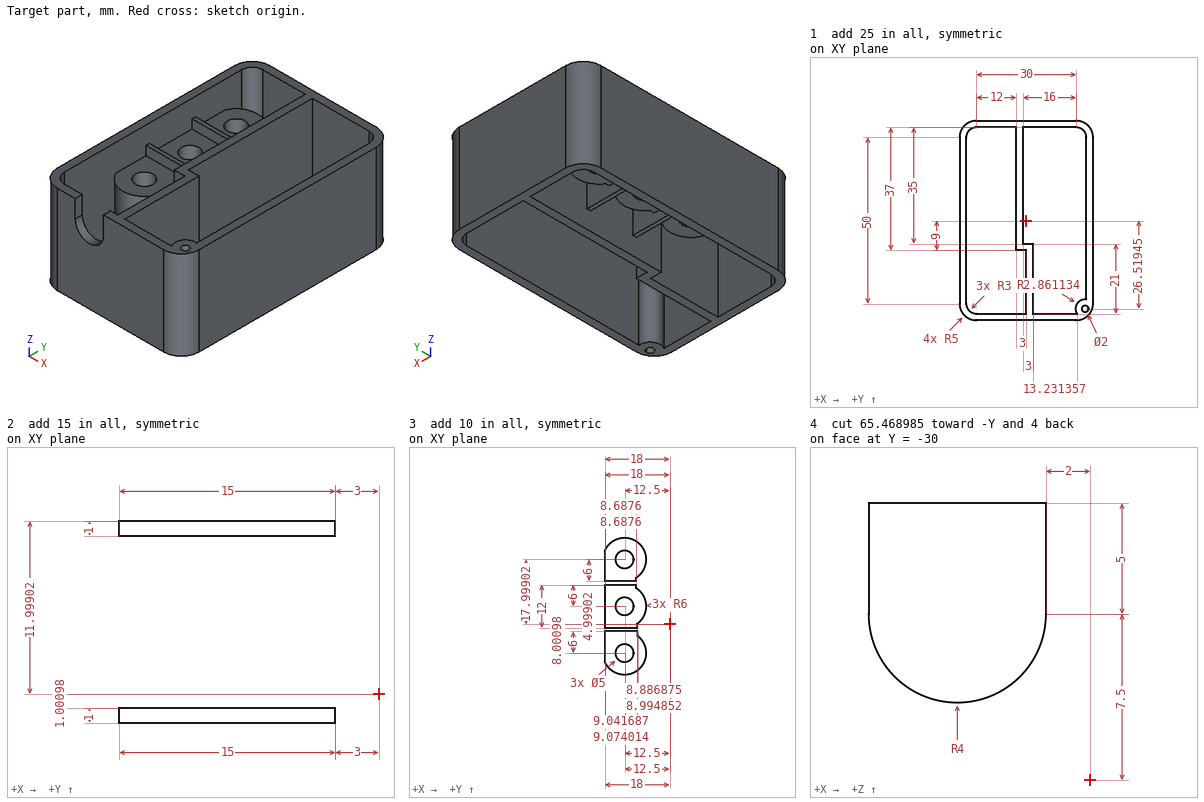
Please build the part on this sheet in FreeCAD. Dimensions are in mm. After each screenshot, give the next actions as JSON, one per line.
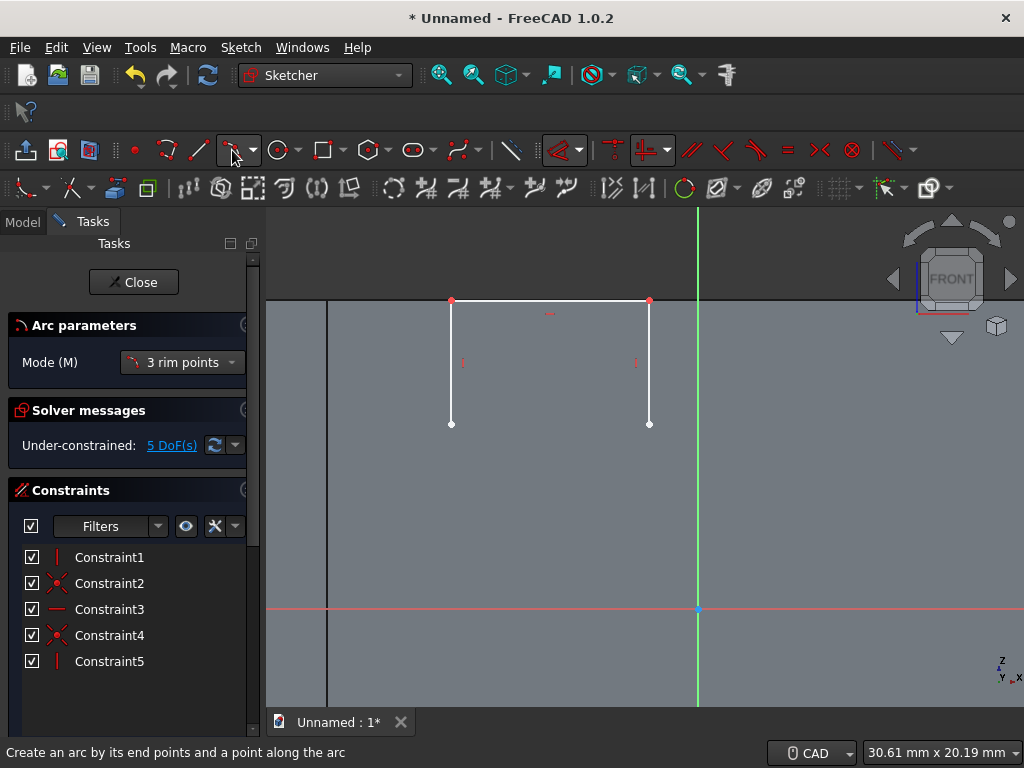
{"action": "left_click", "coordinate": [451, 425]}
{"action": "left_click", "coordinate": [649, 425]}
{"action": "left_click", "coordinate": [550, 523]}
{"action": "key", "text": "Escape"}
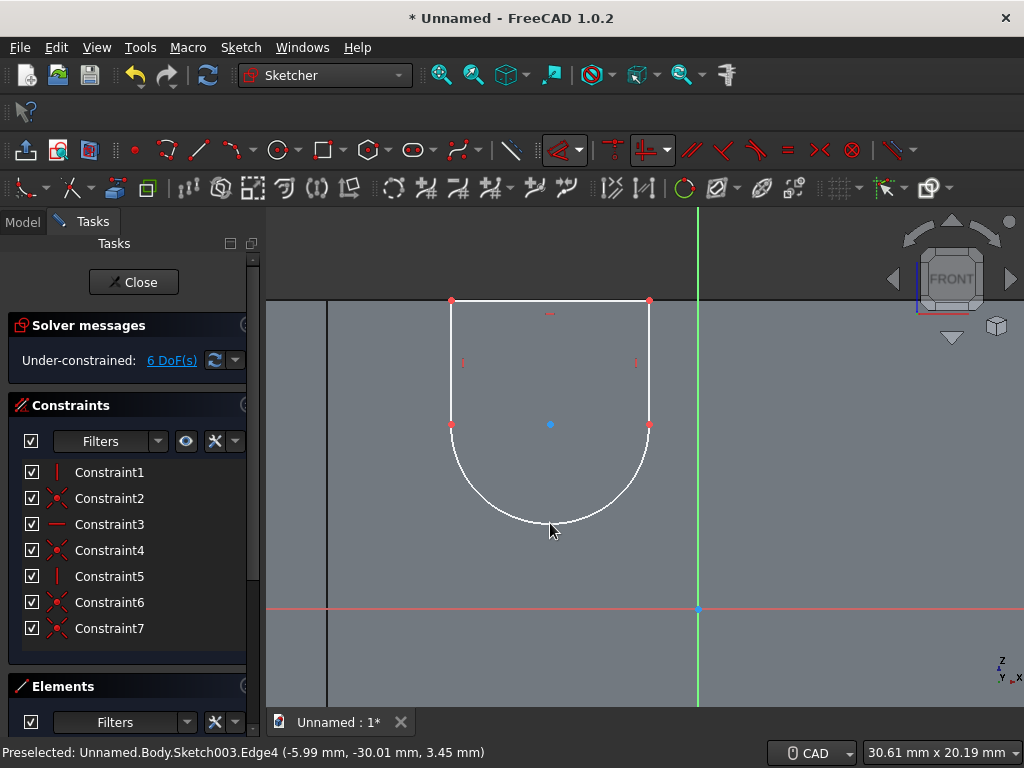
{"action": "left_click", "coordinate": [649, 388]}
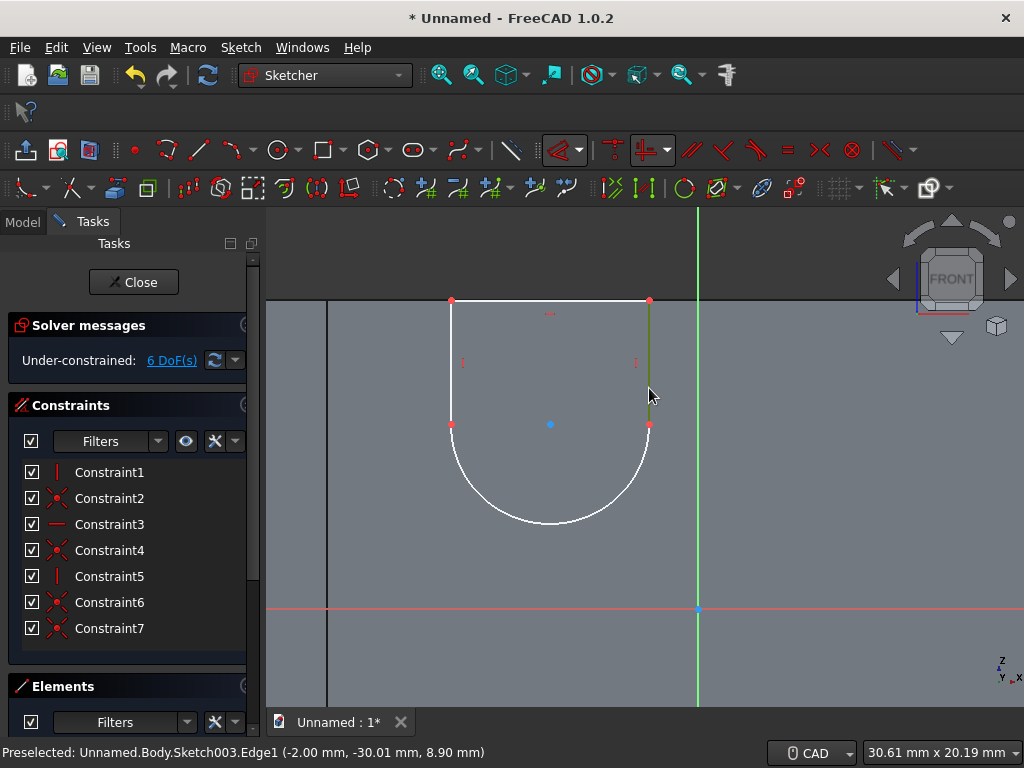
{"action": "left_click", "coordinate": [492, 505]}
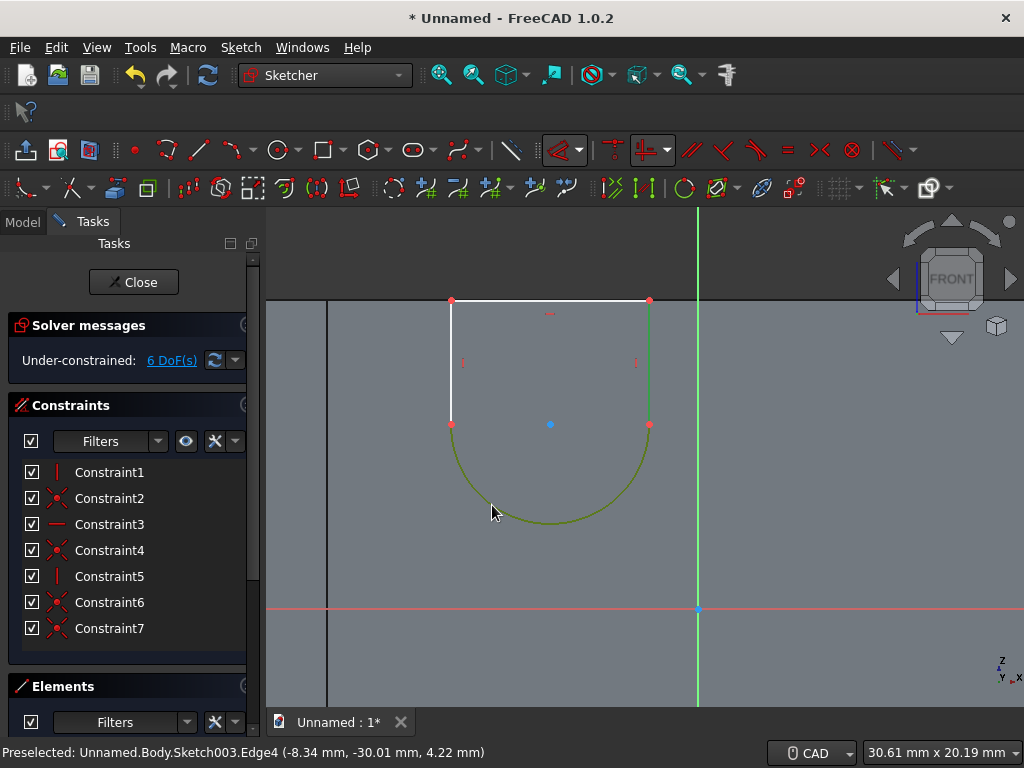
{"action": "left_click", "coordinate": [756, 150]}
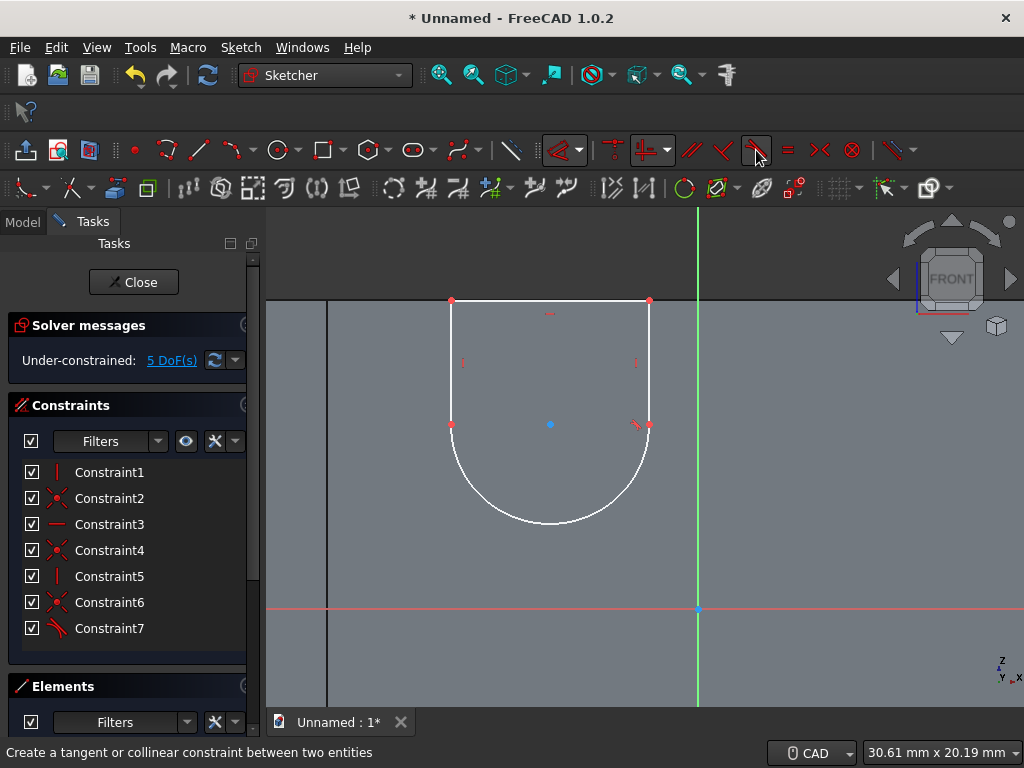
{"action": "left_click", "coordinate": [451, 338]}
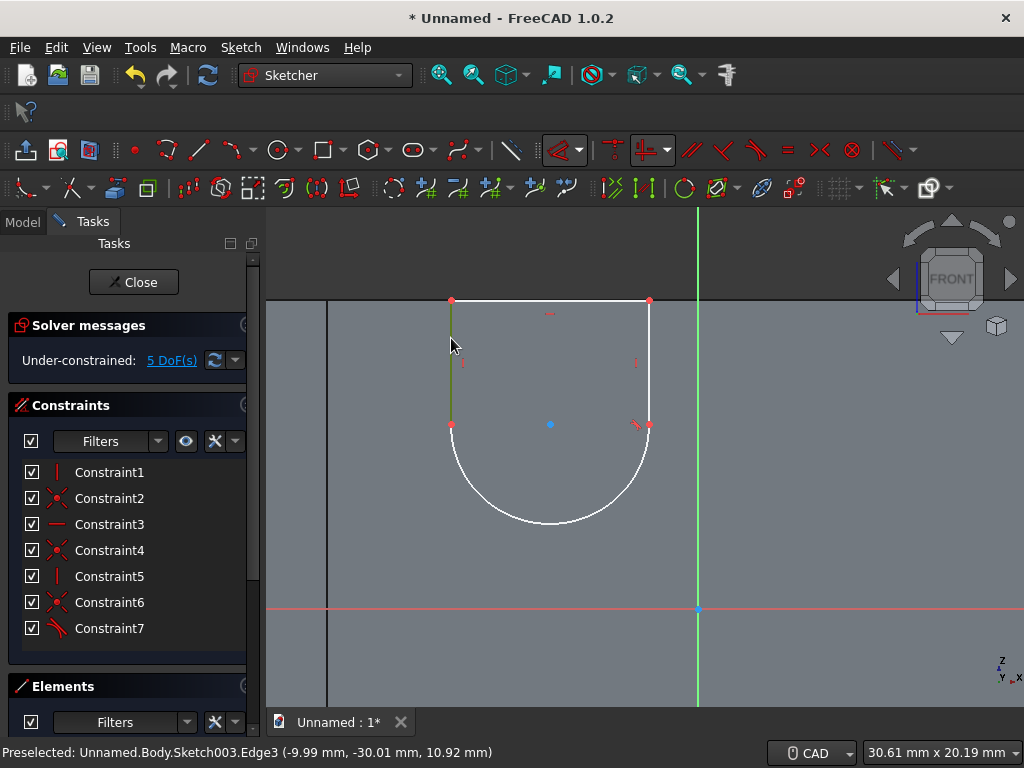
{"action": "left_click", "coordinate": [492, 505]}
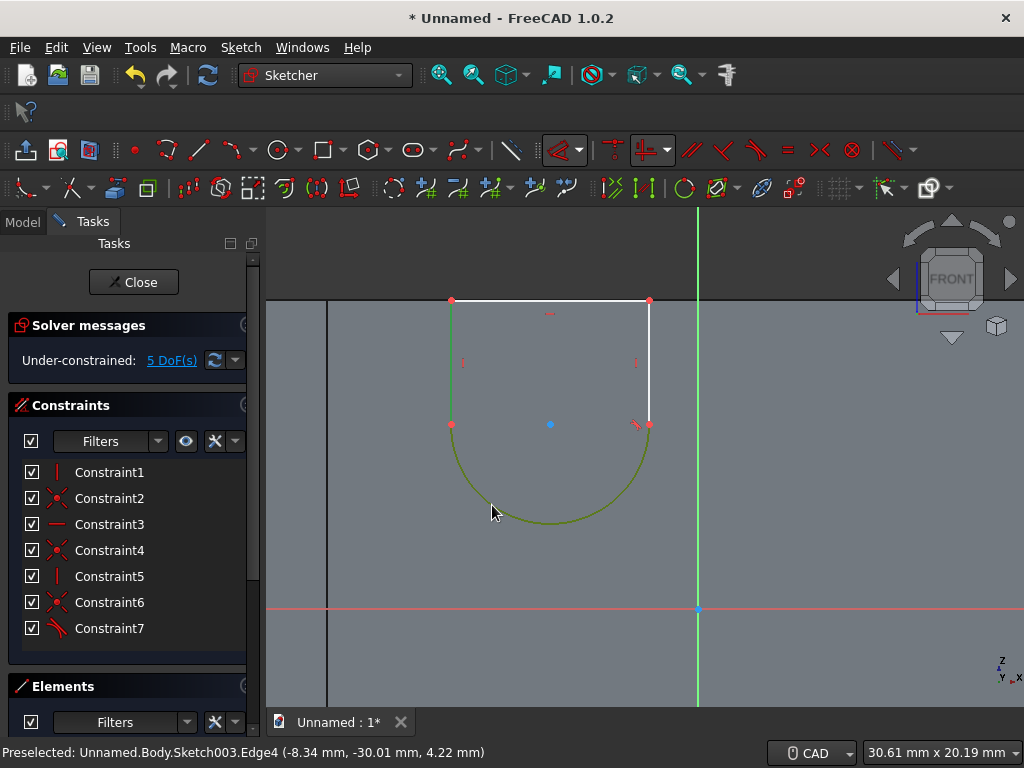
{"action": "left_click", "coordinate": [756, 150]}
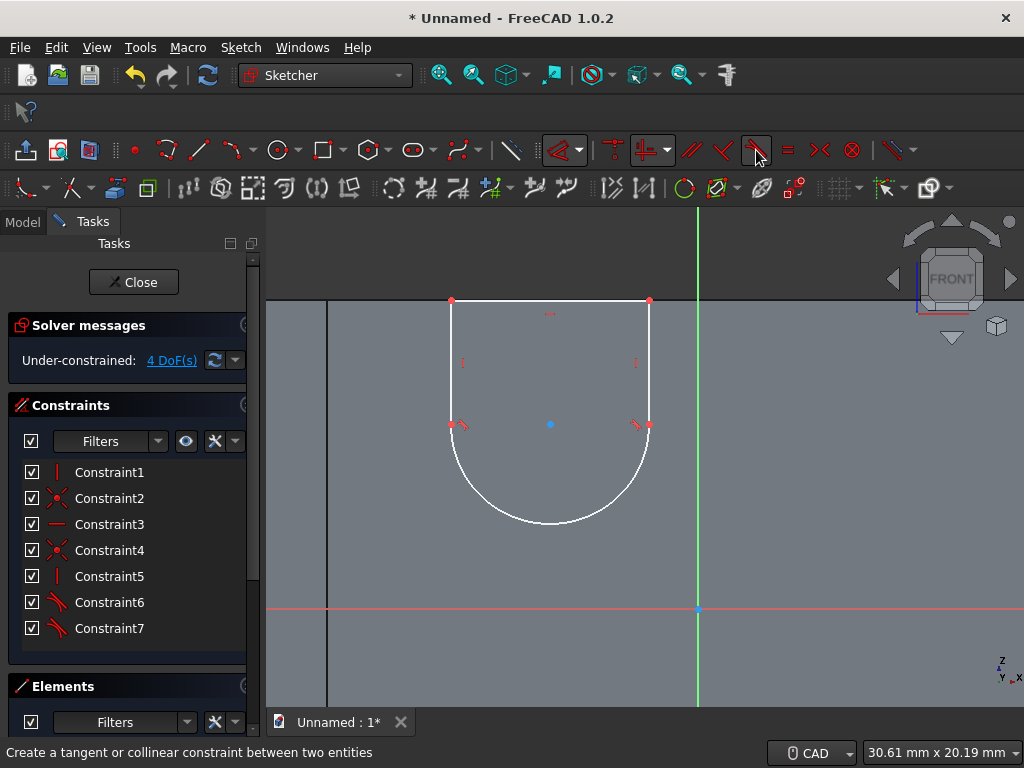
{"action": "left_click", "coordinate": [492, 505]}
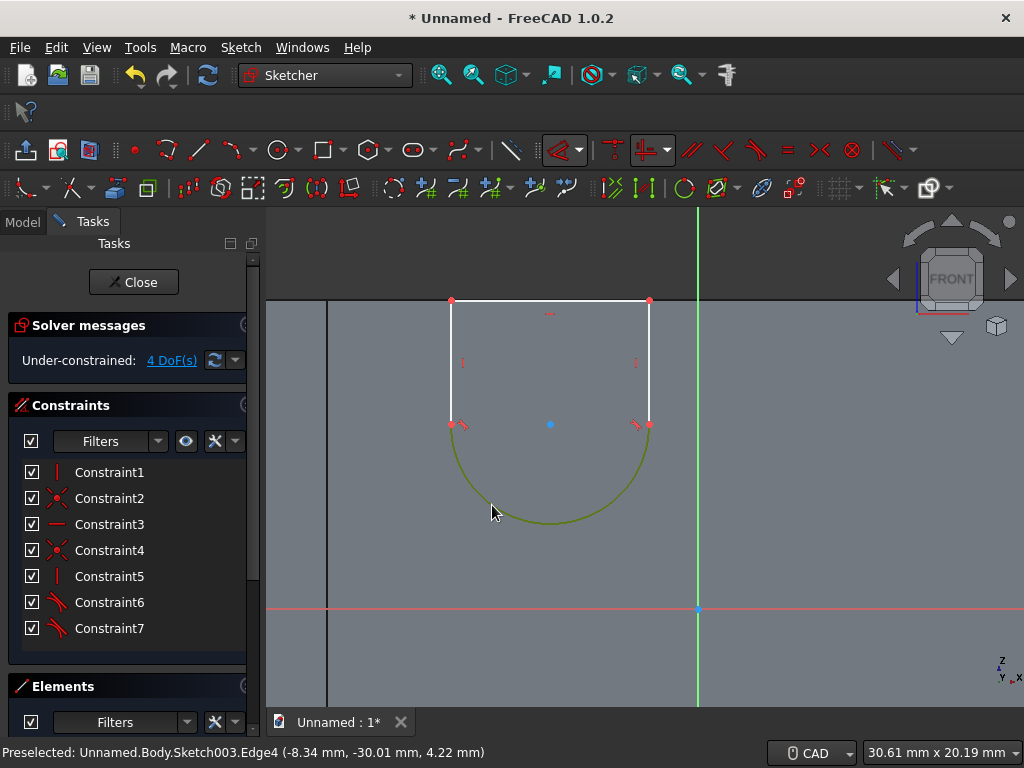
{"action": "key", "text": "k r"}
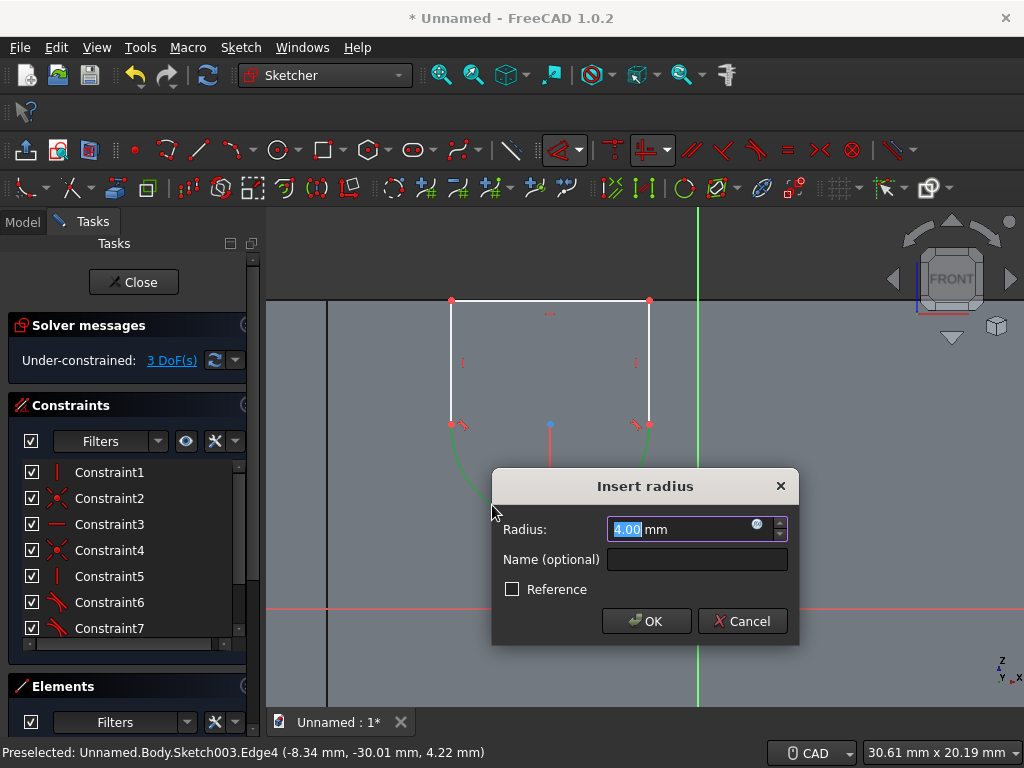
{"action": "type", "text": "4"}
{"action": "key", "text": "Return"}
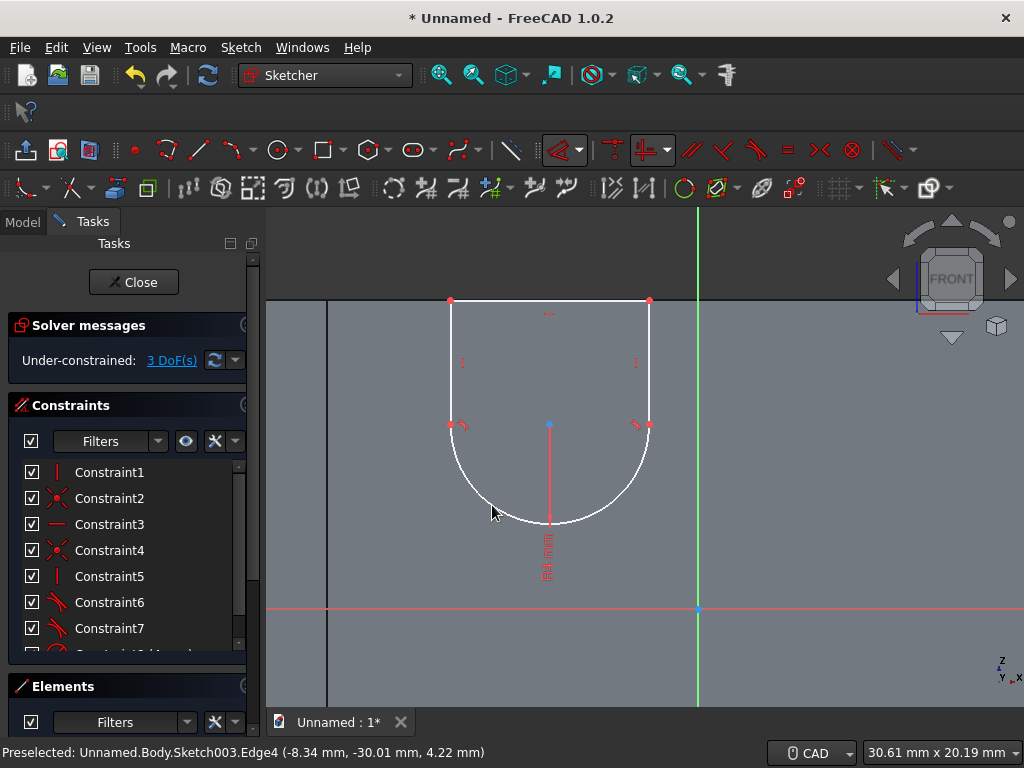
{"action": "left_click", "coordinate": [649, 388]}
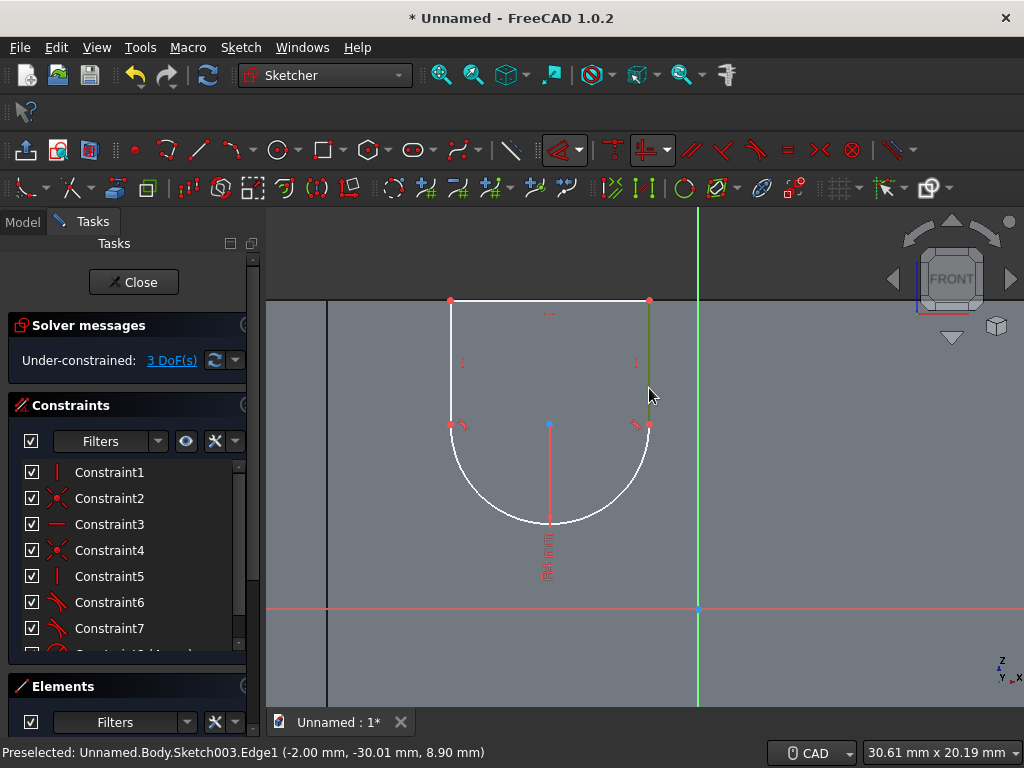
{"action": "left_click", "coordinate": [582, 150]}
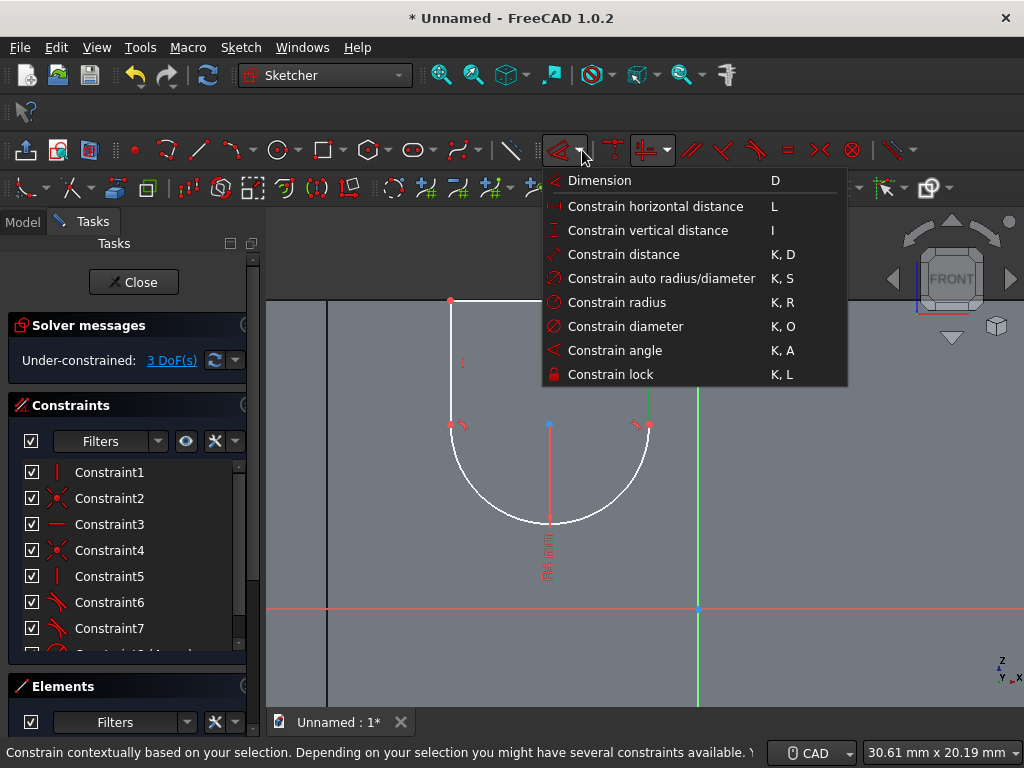
{"action": "left_click", "coordinate": [695, 230]}